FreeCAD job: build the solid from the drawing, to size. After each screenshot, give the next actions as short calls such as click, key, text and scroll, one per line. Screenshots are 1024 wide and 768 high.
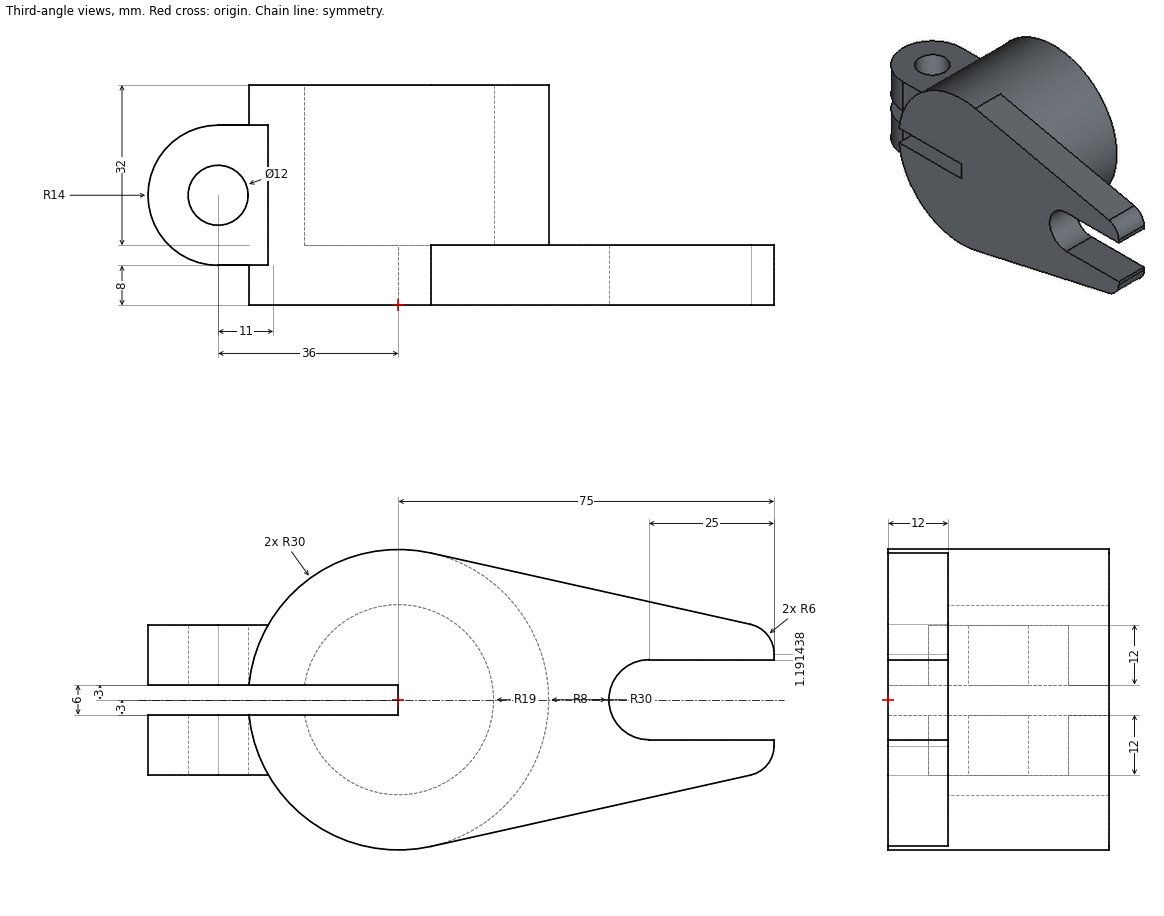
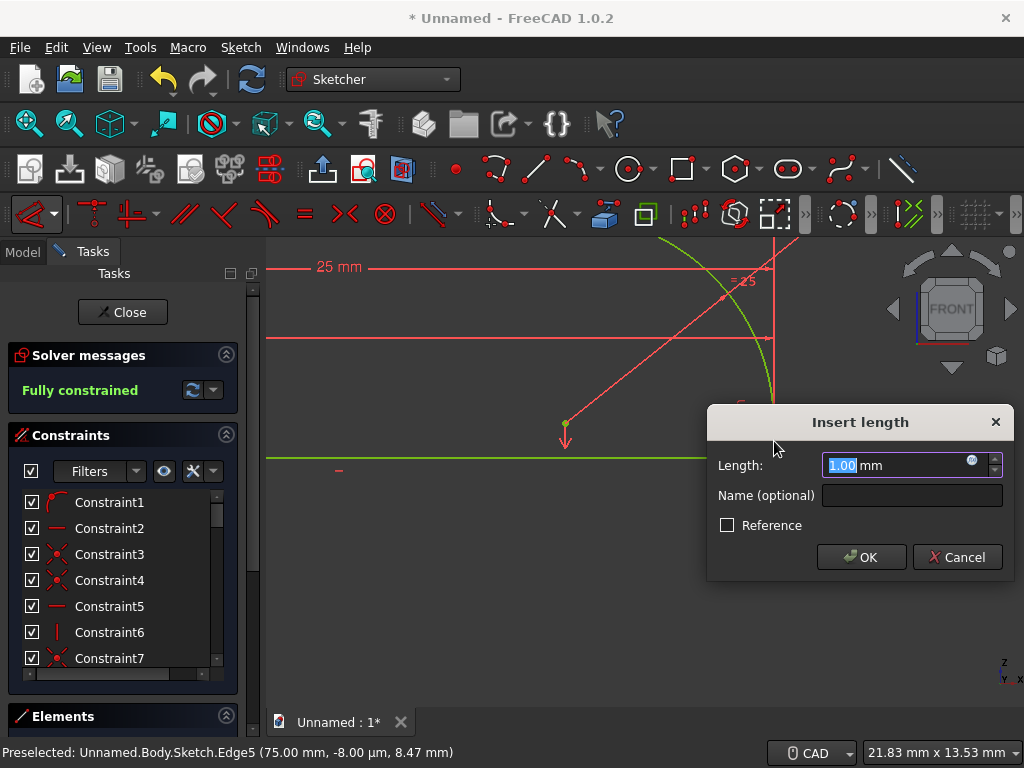
text(1.191438)
key(Return)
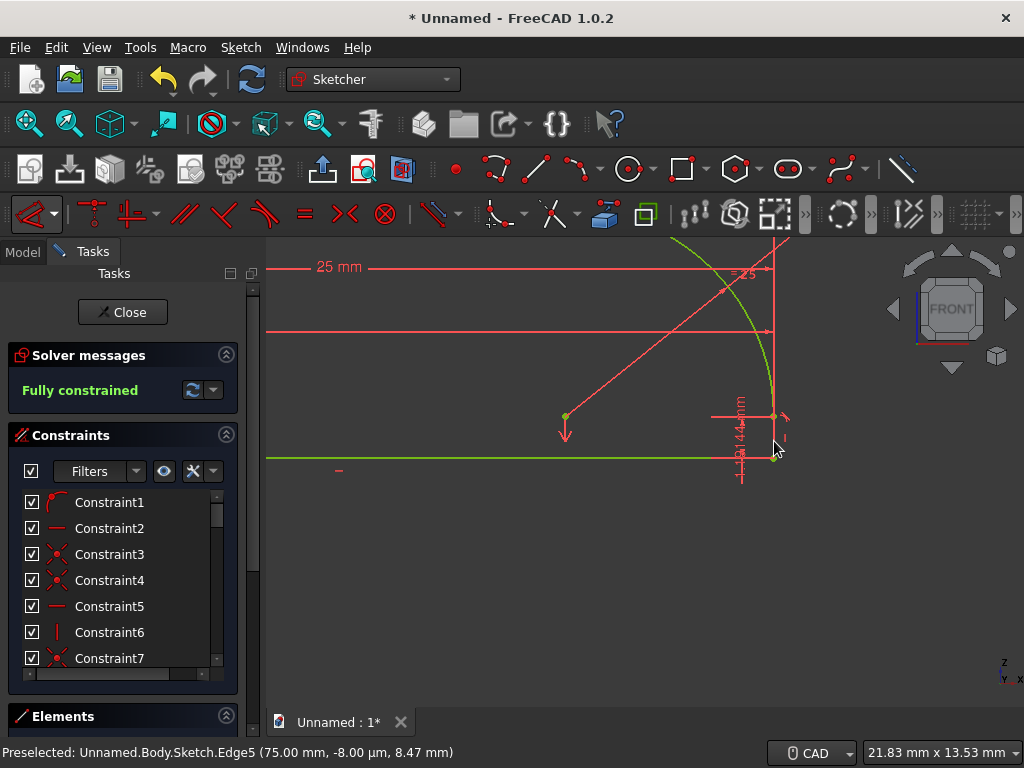
click(123, 312)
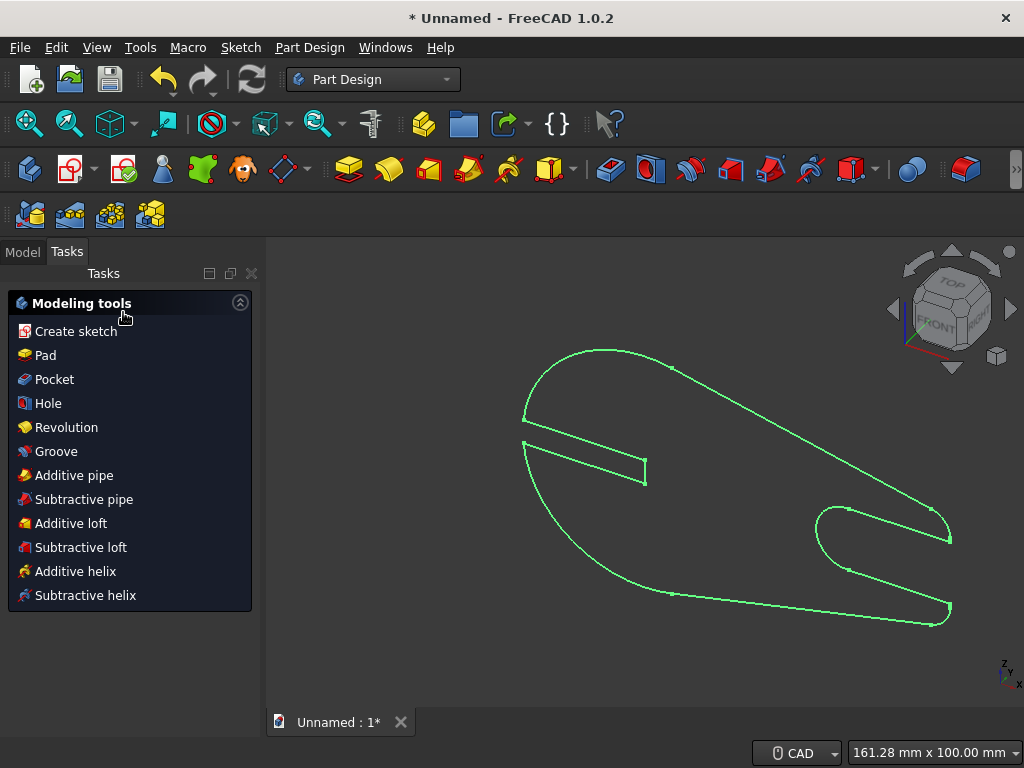
click(350, 170)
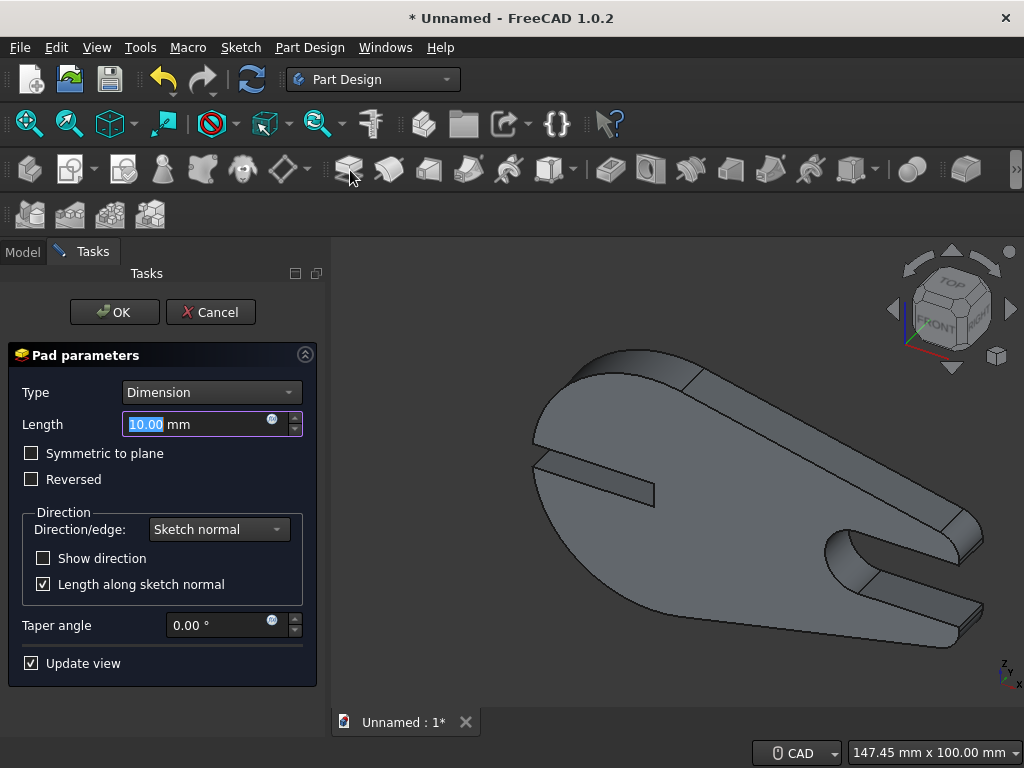
text(12)
key(Tab)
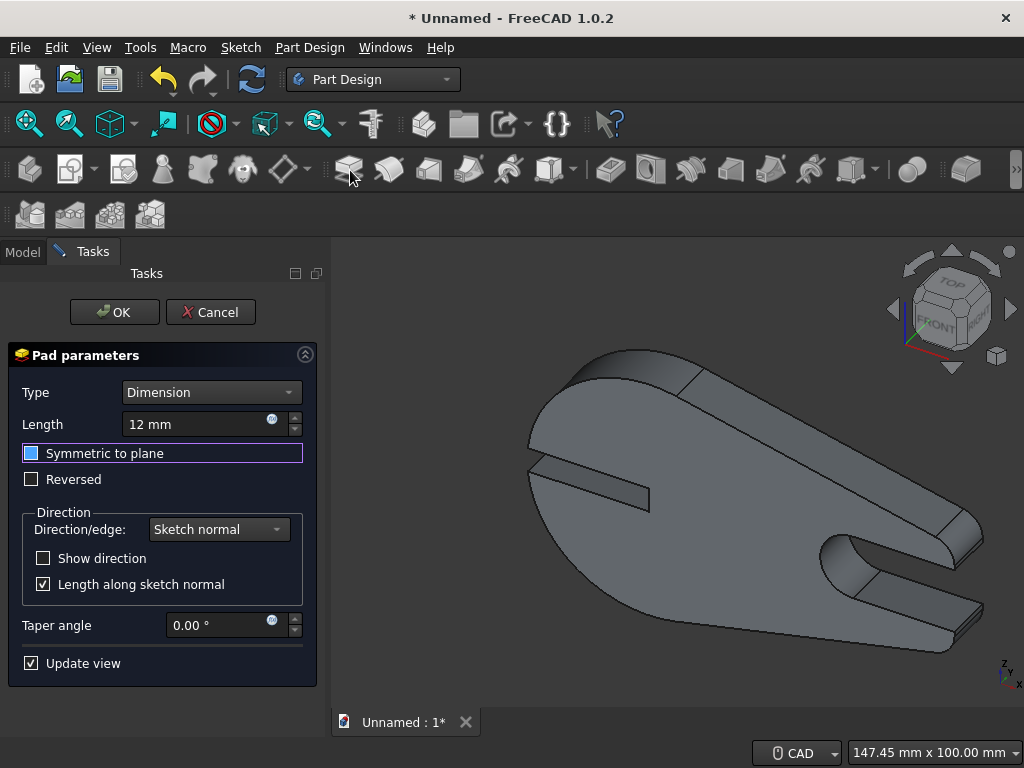
click(30, 479)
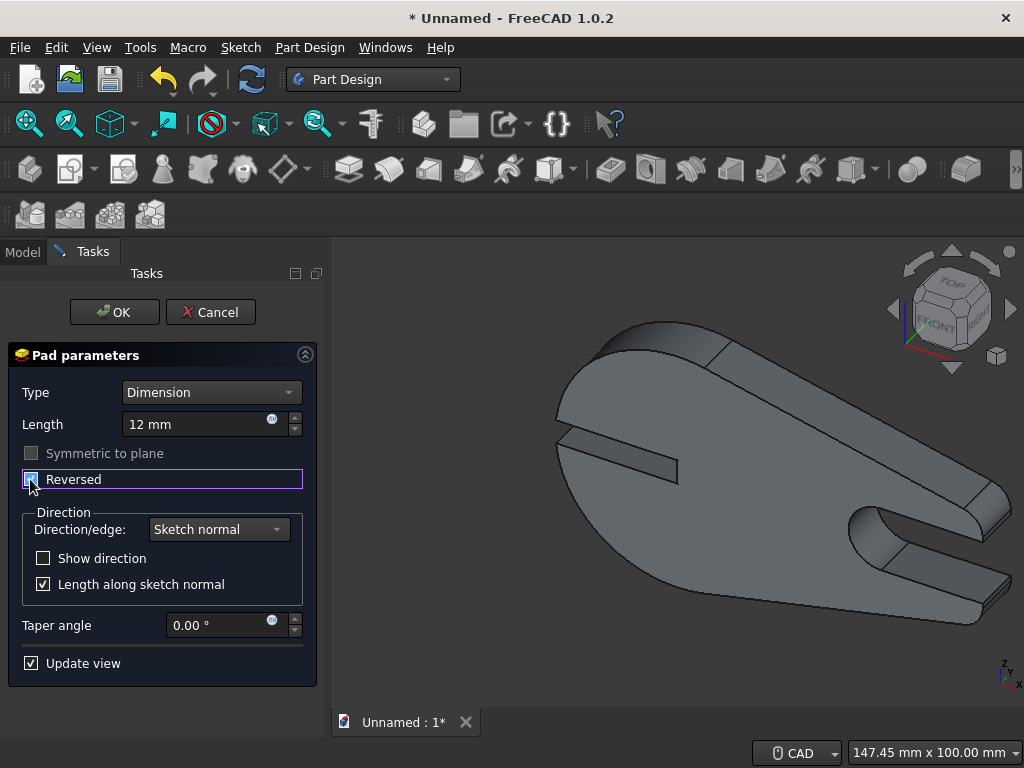
click(115, 312)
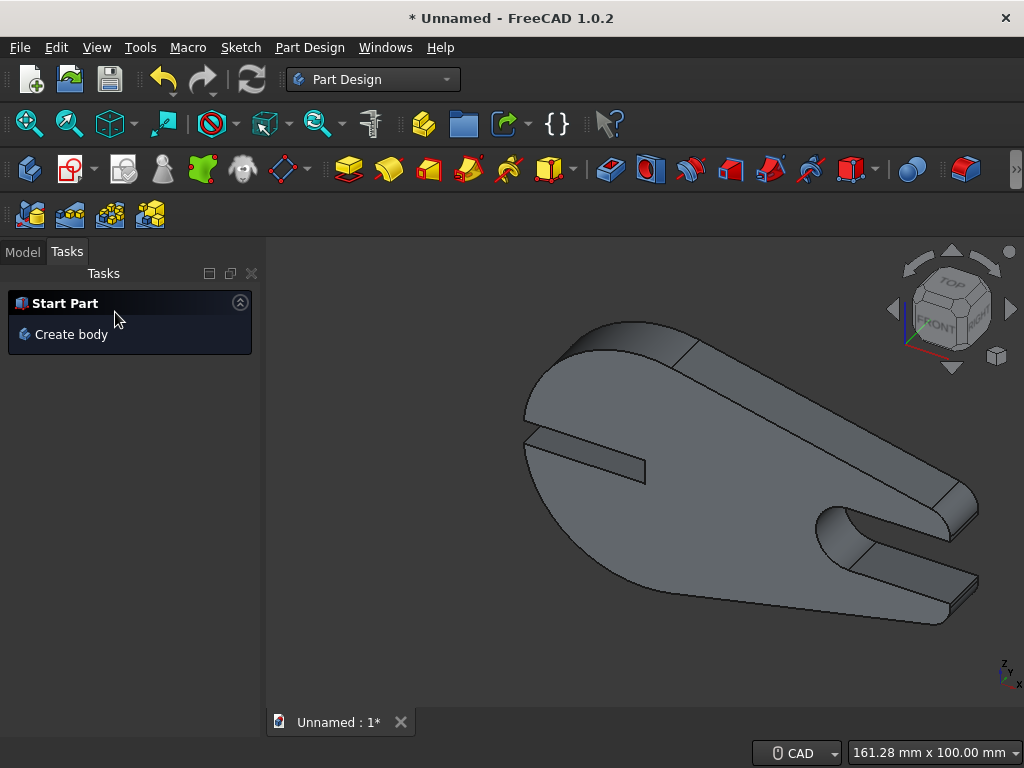
key(4)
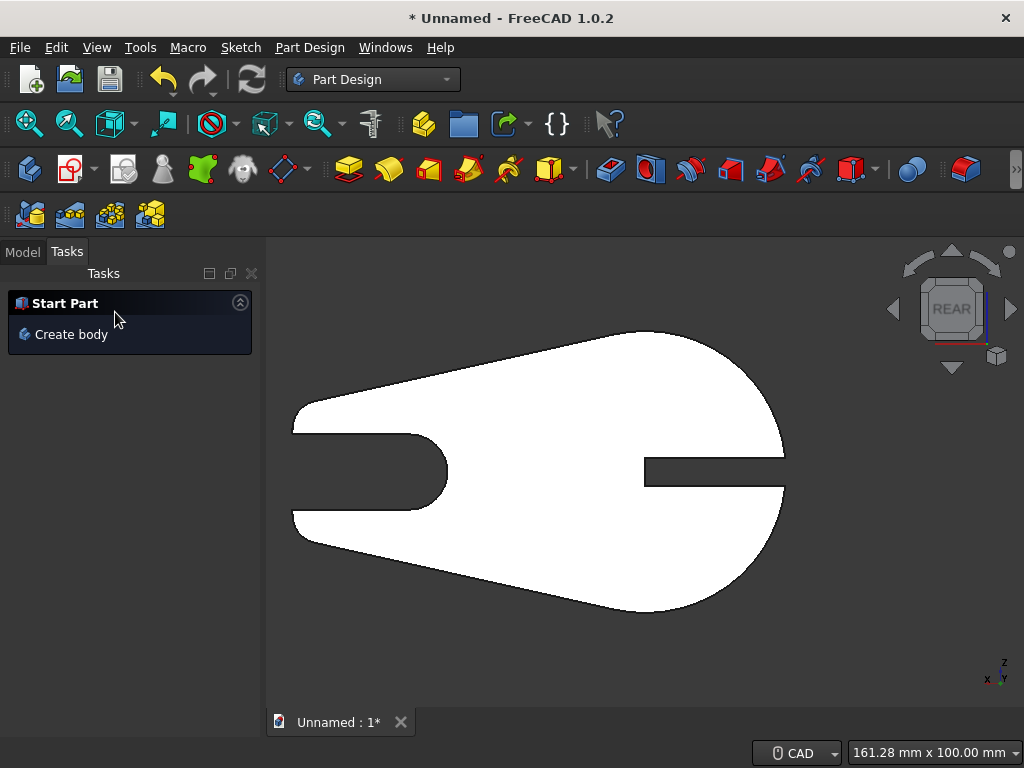
click(539, 471)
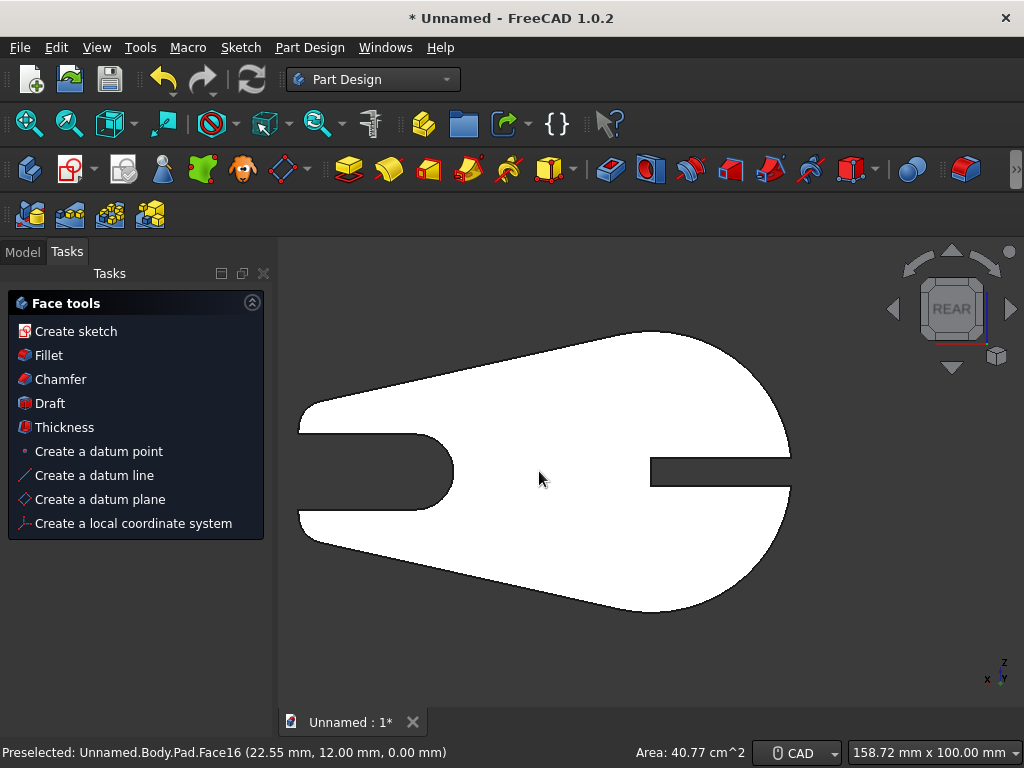
click(70, 170)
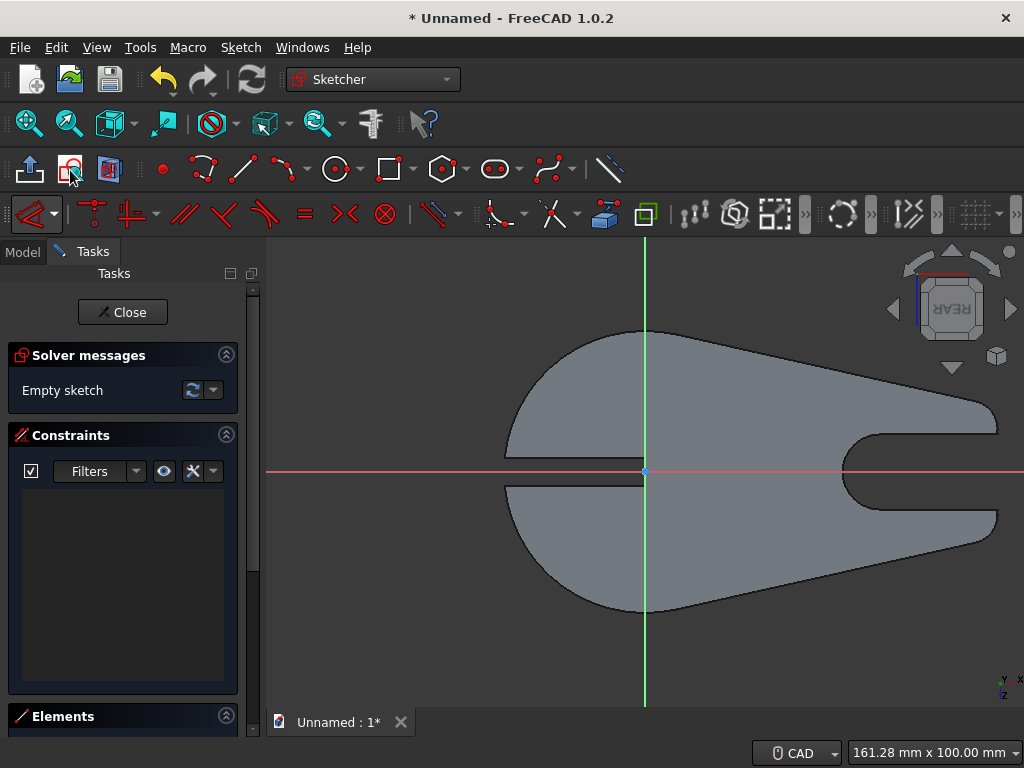
scroll(785, 472, up, 2)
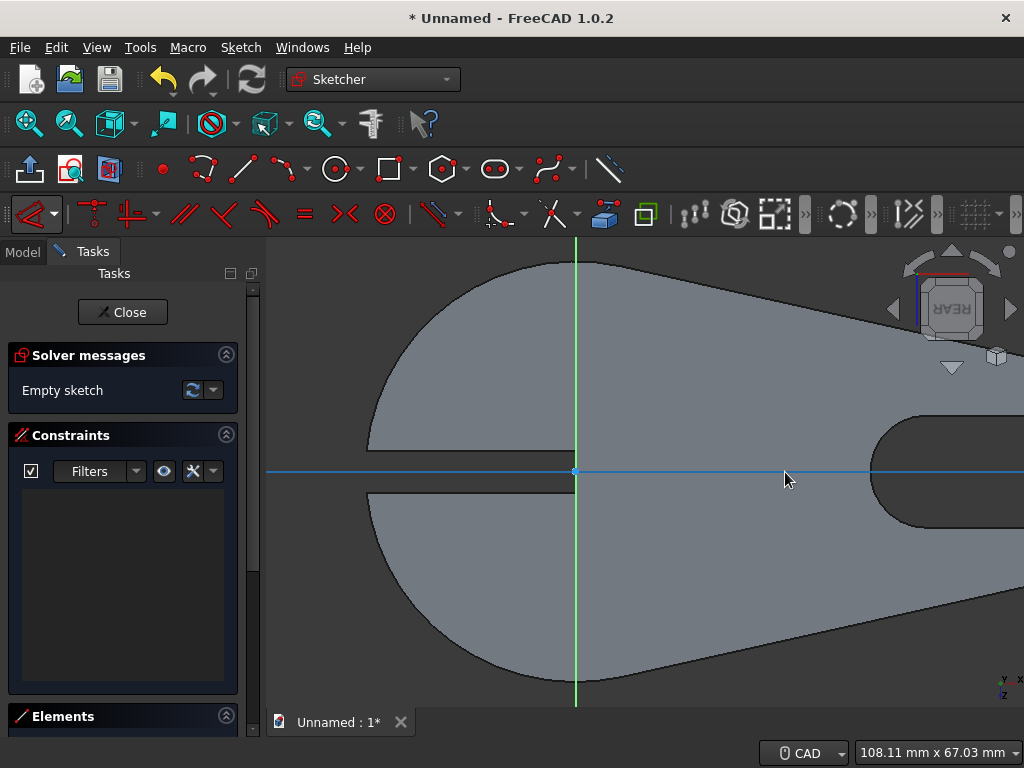
key(g)
key(l)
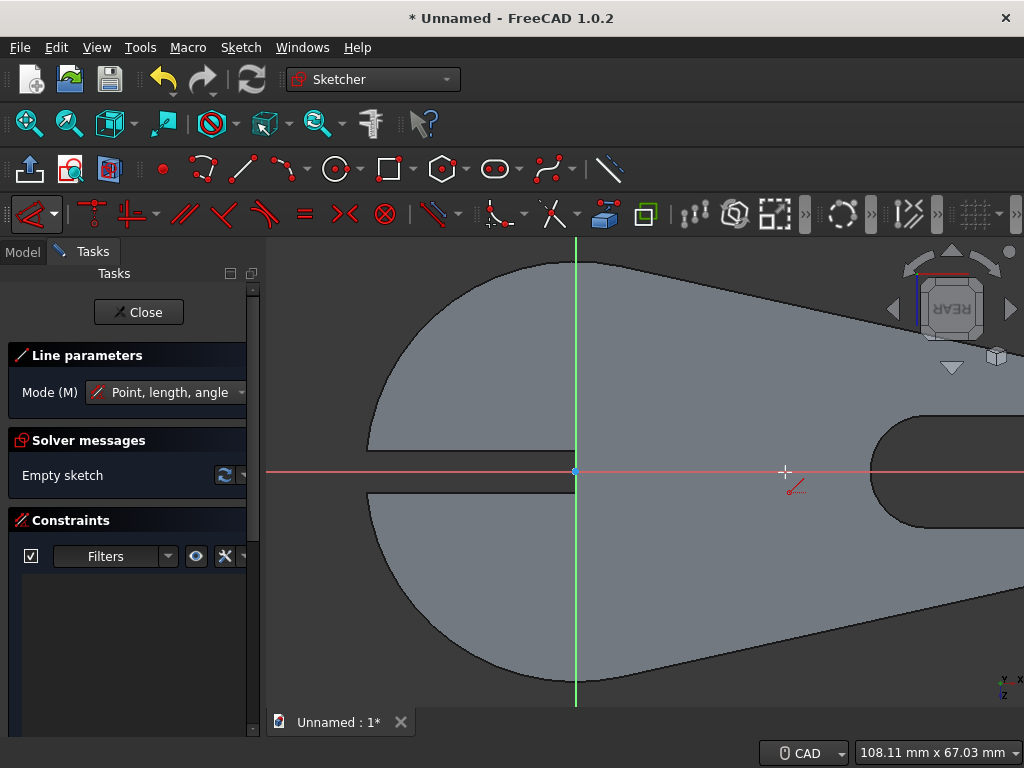
click(367, 451)
click(444, 451)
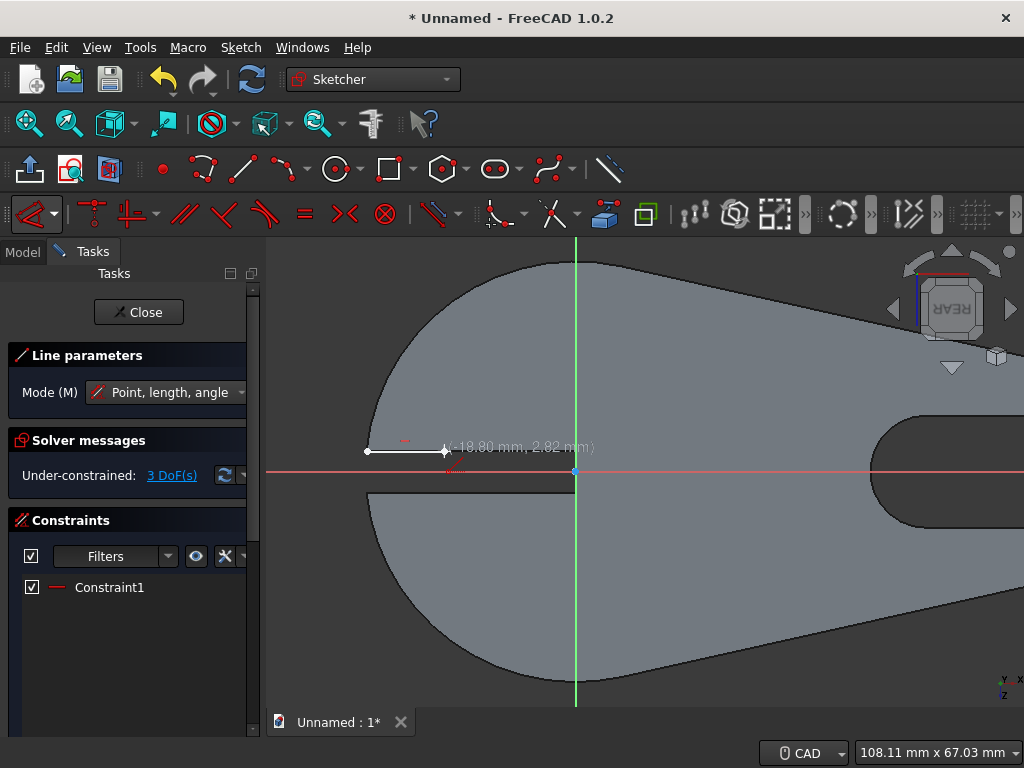
click(444, 493)
click(367, 493)